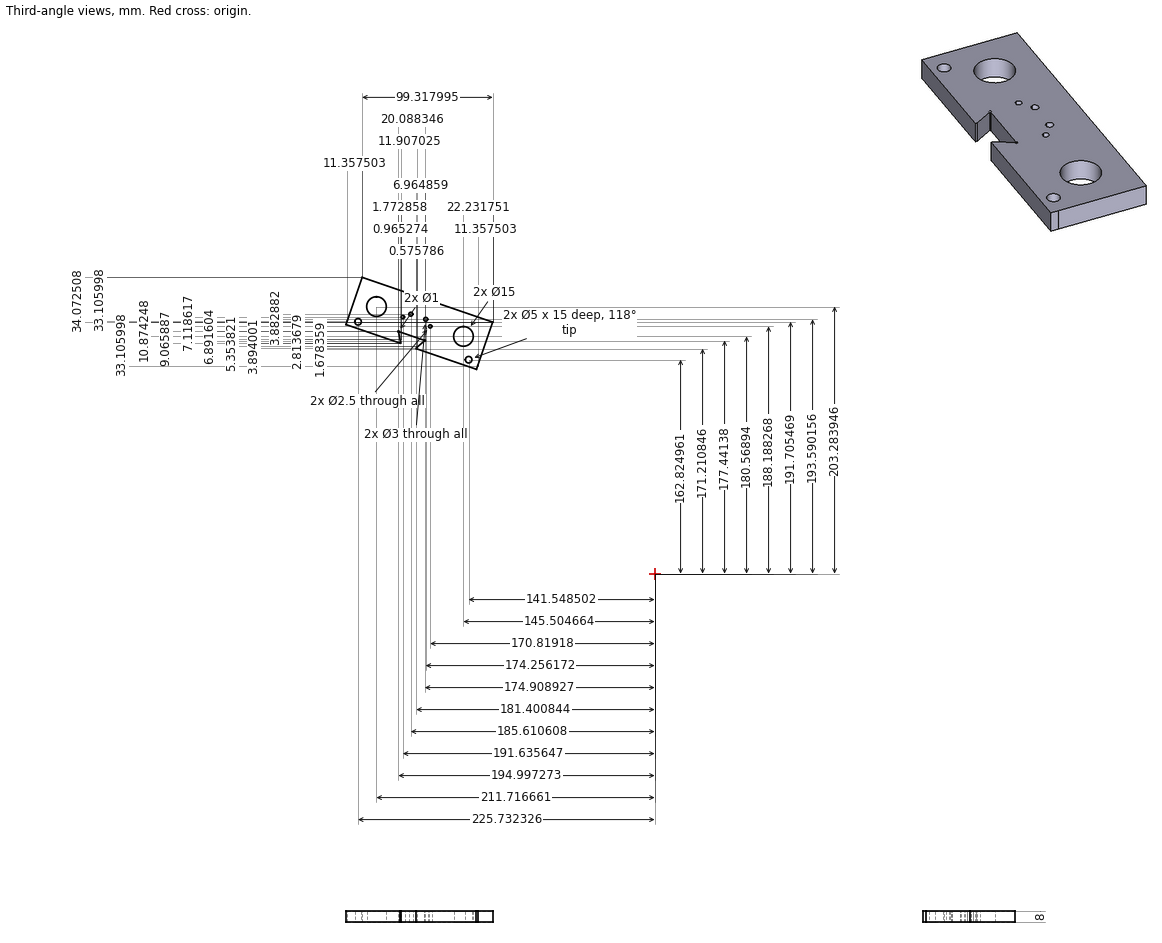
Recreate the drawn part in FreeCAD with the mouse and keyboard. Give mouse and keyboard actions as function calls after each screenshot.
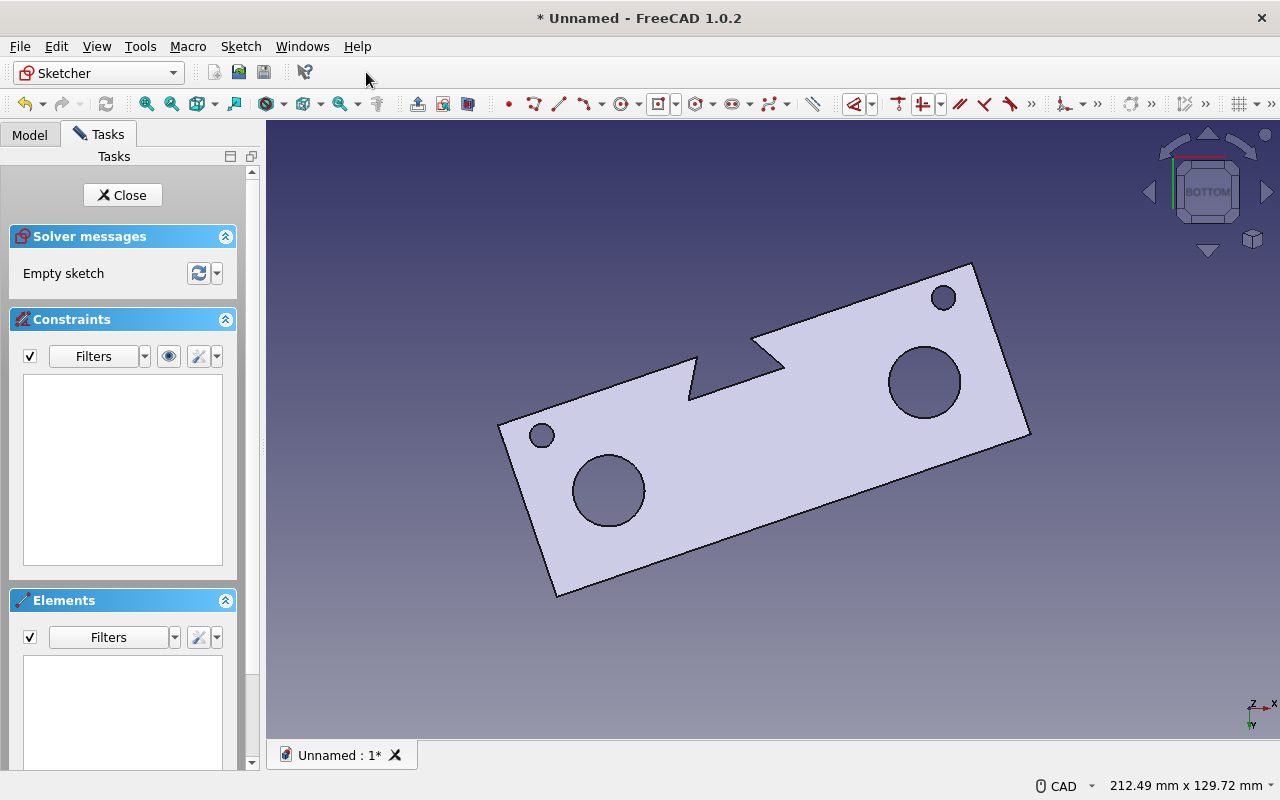
scroll(767, 437, up, 8)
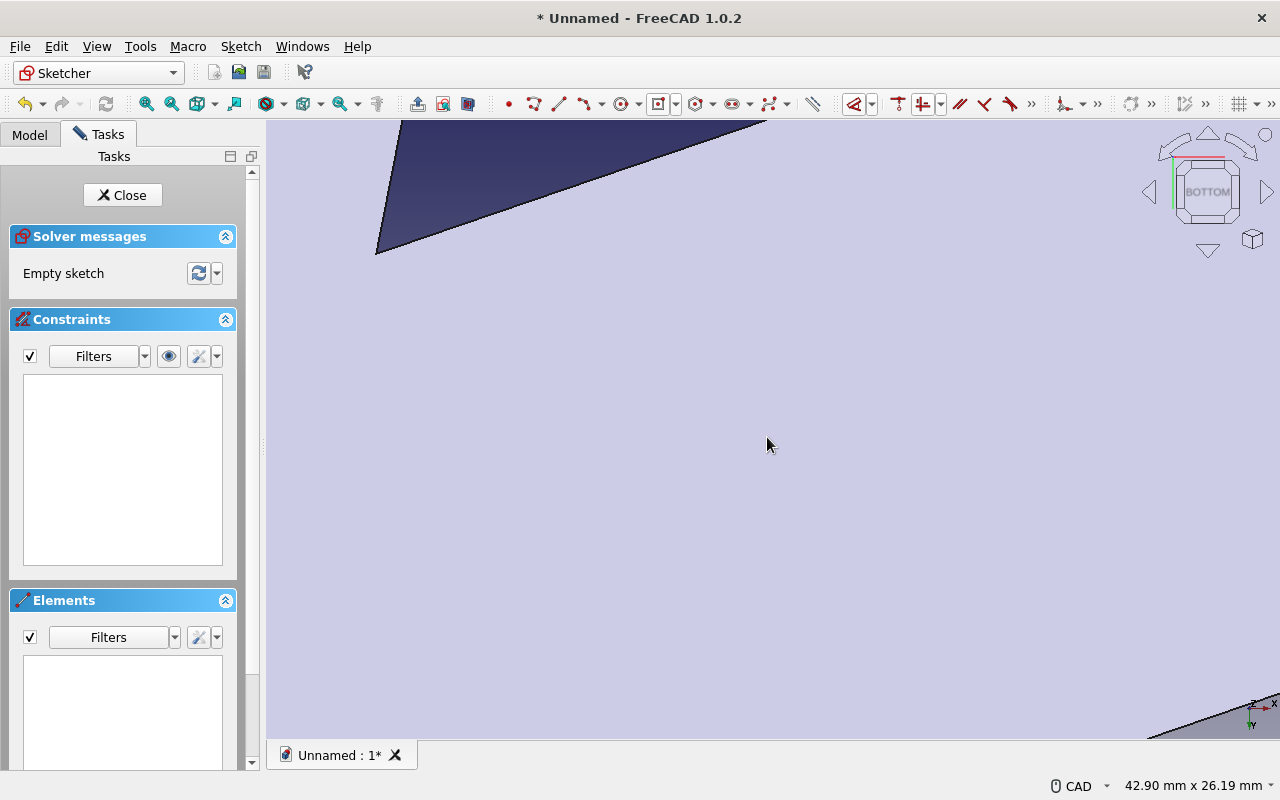
click(620, 104)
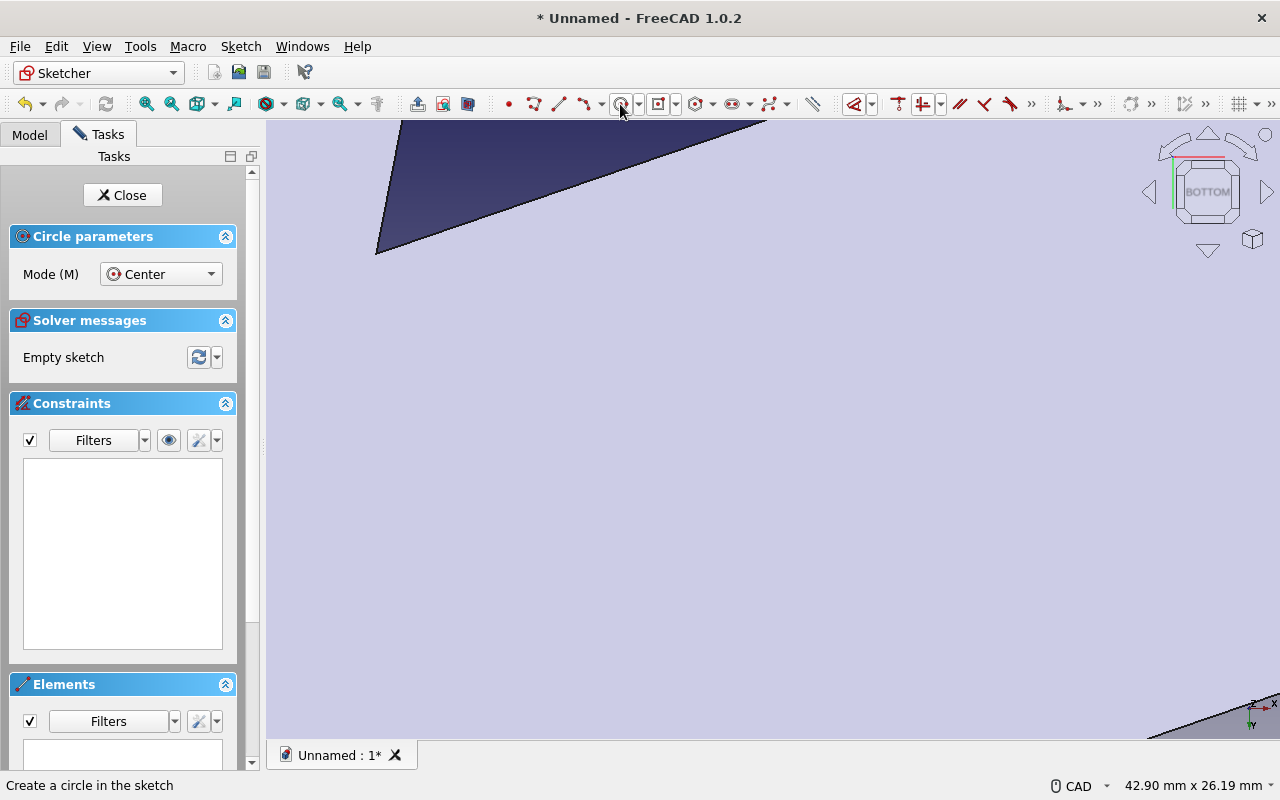
click(948, 345)
click(969, 324)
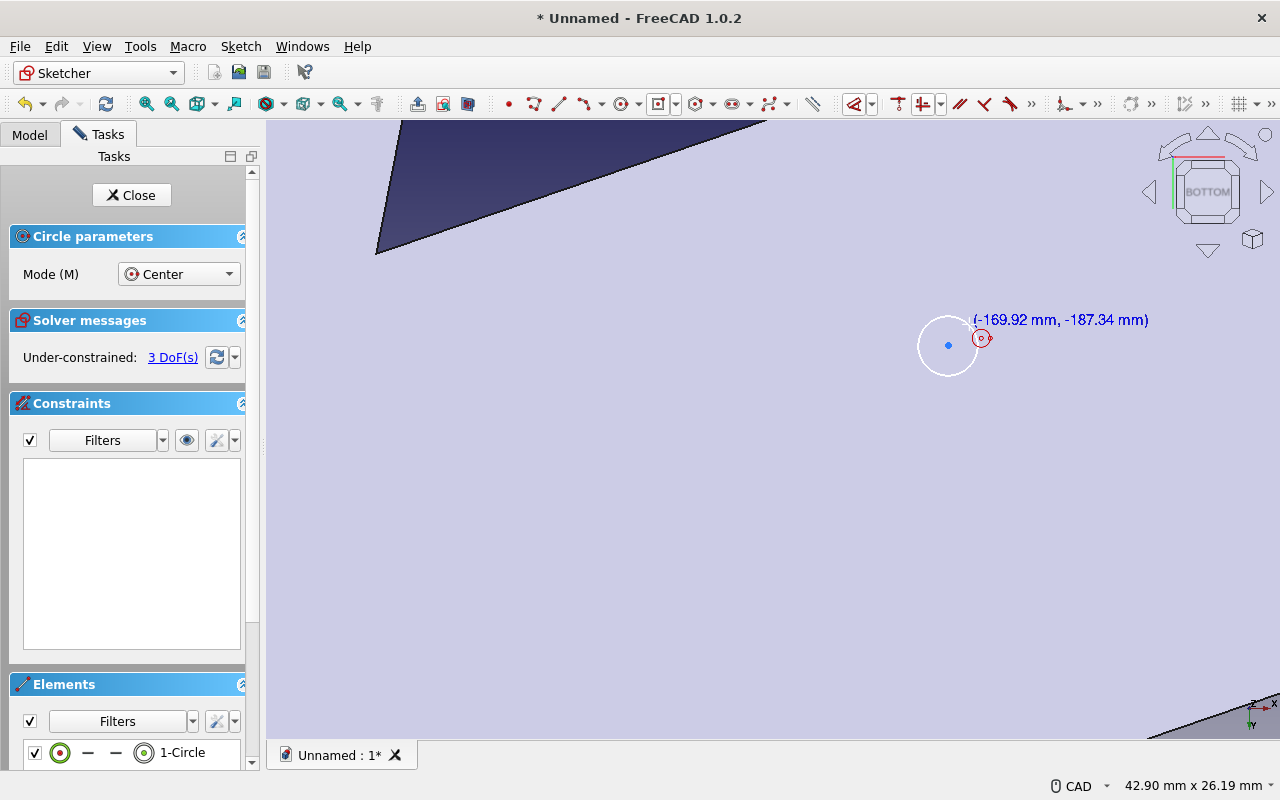
click(456, 513)
click(477, 492)
key(Escape)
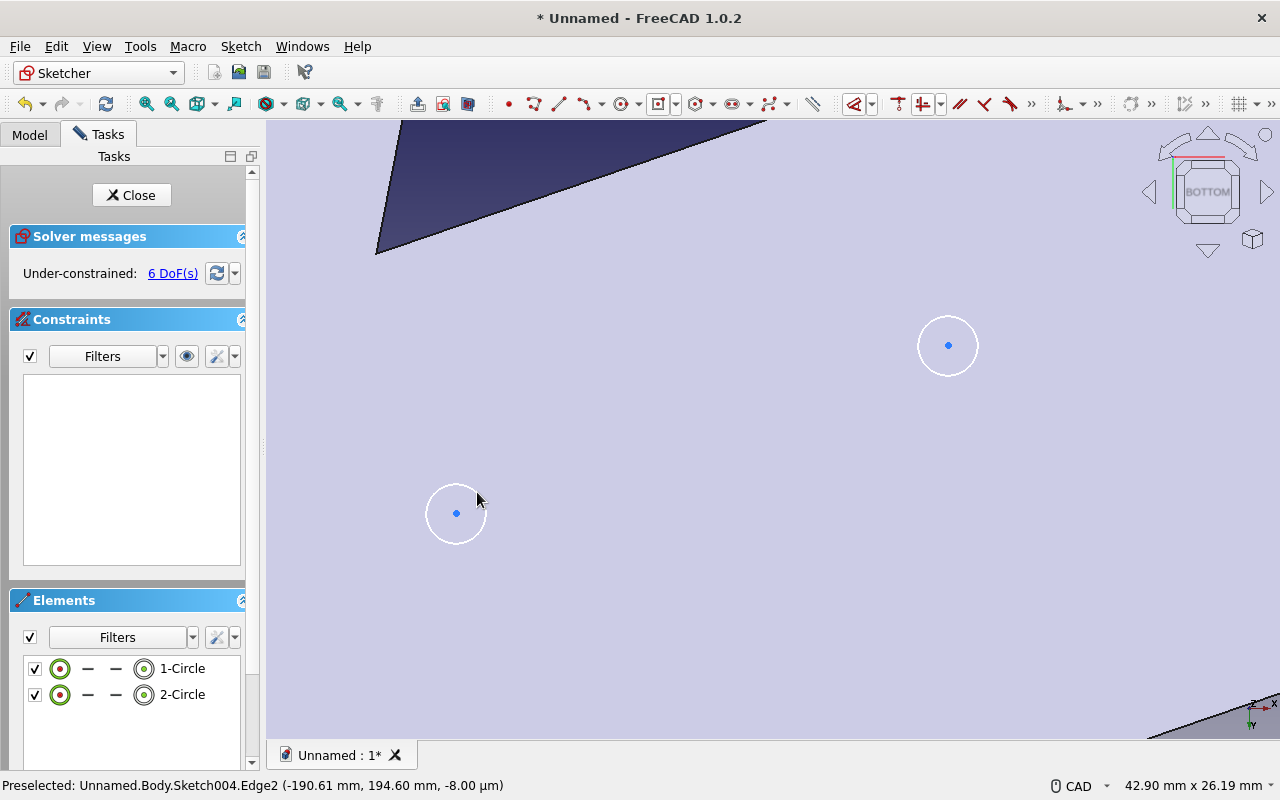
click(969, 325)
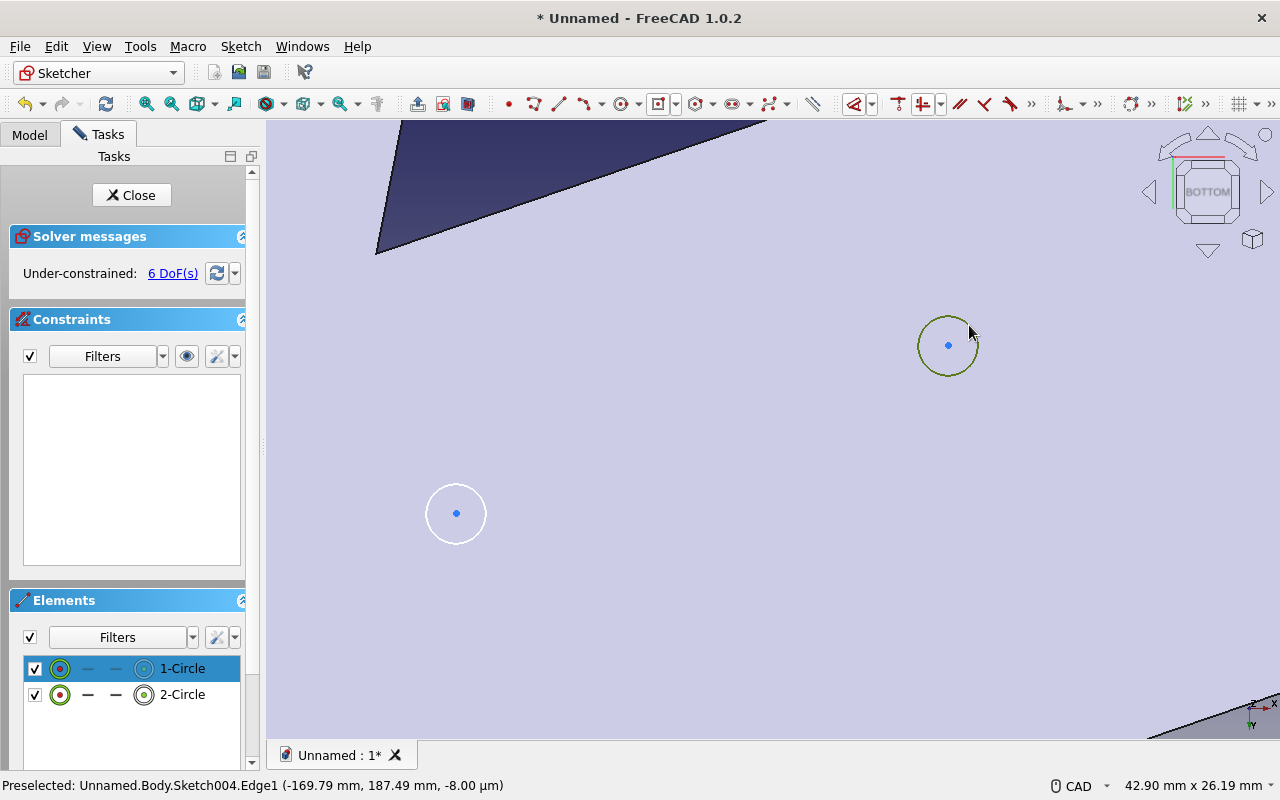
click(477, 493)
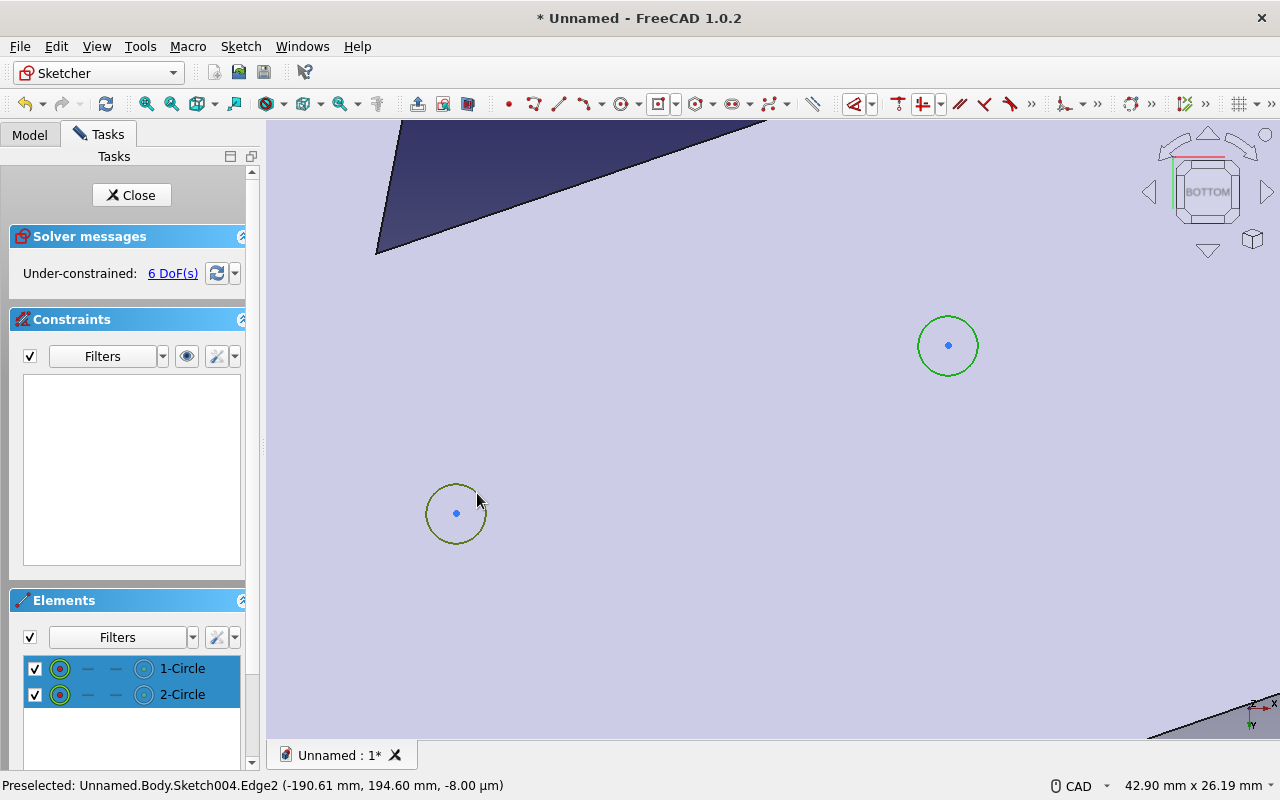
key(e)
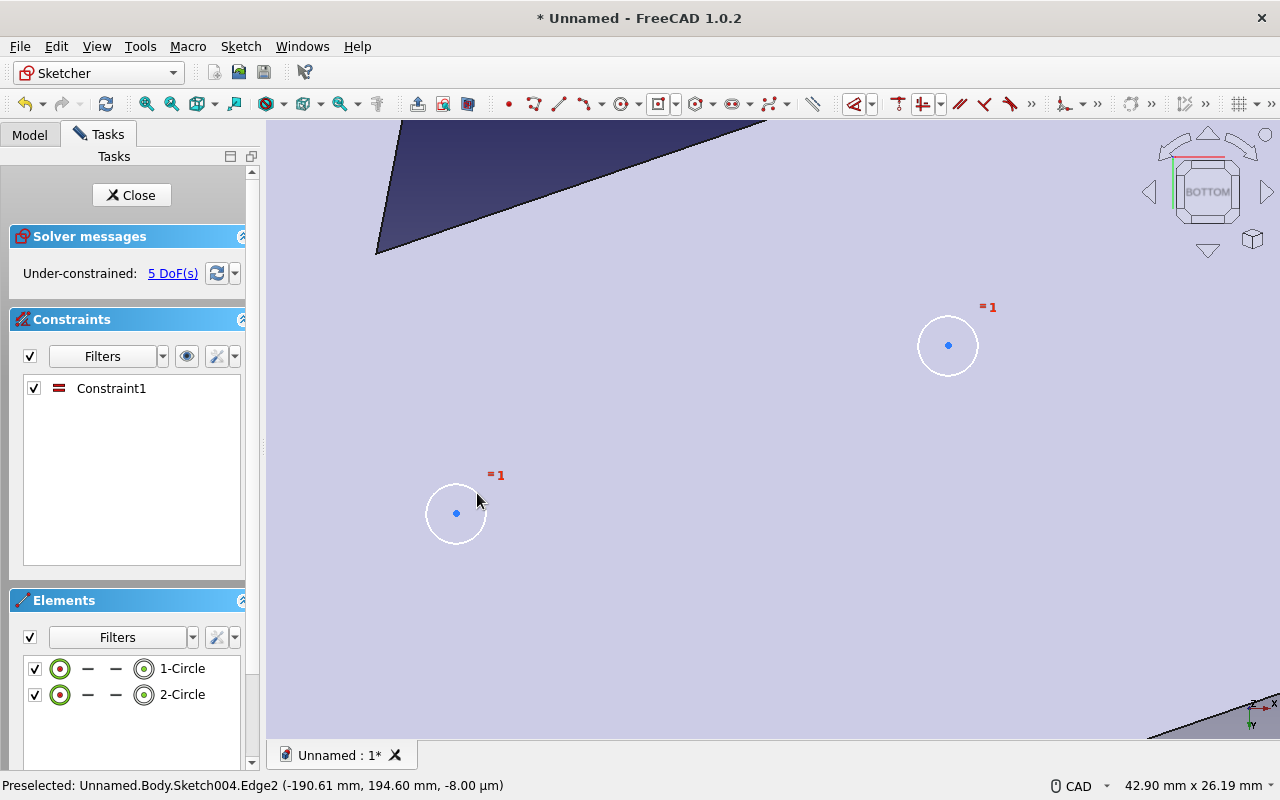
click(969, 325)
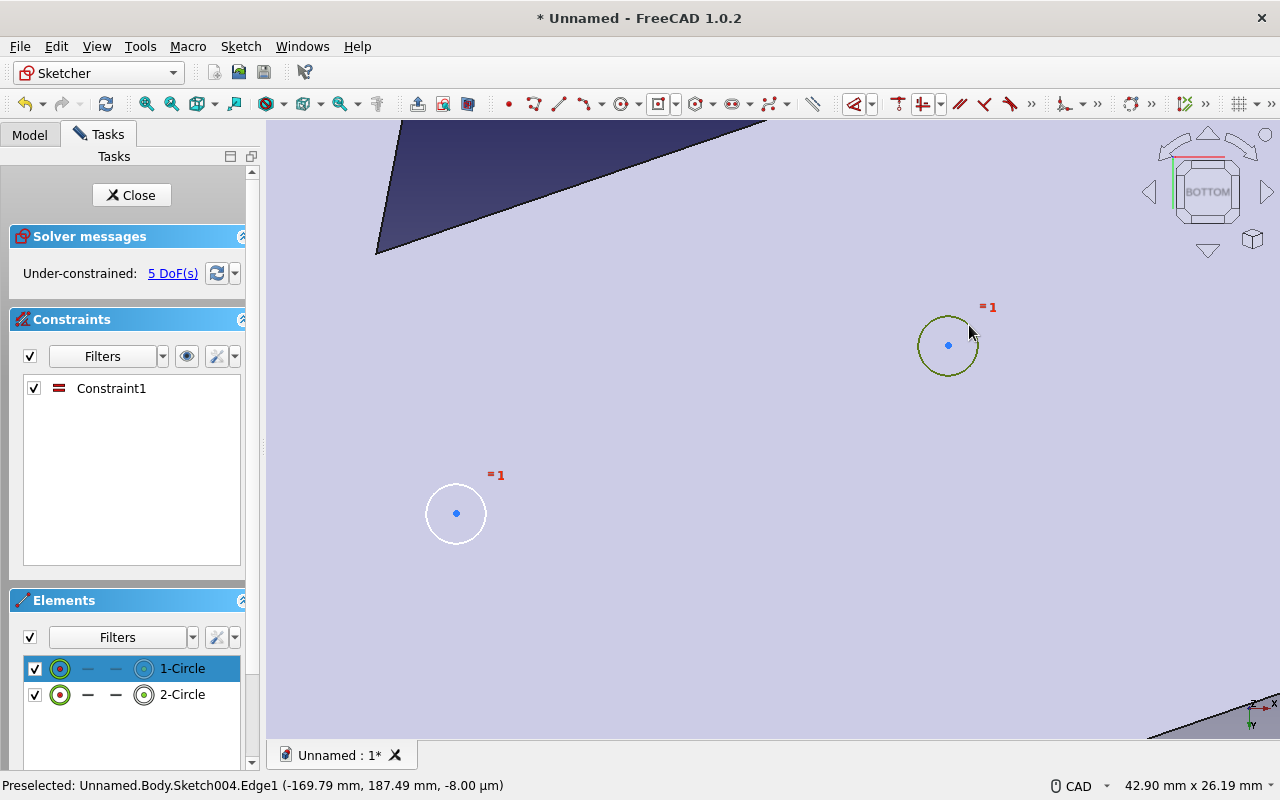
click(872, 104)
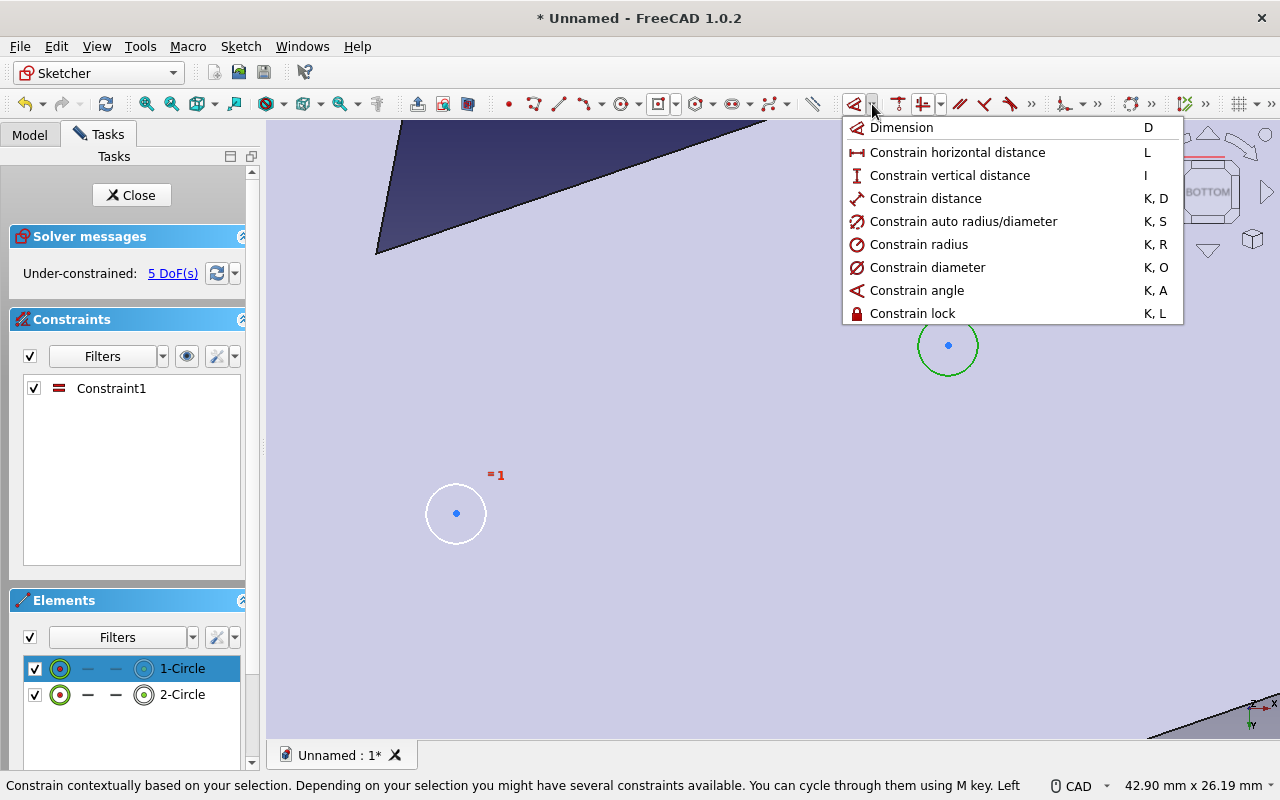
click(1013, 268)